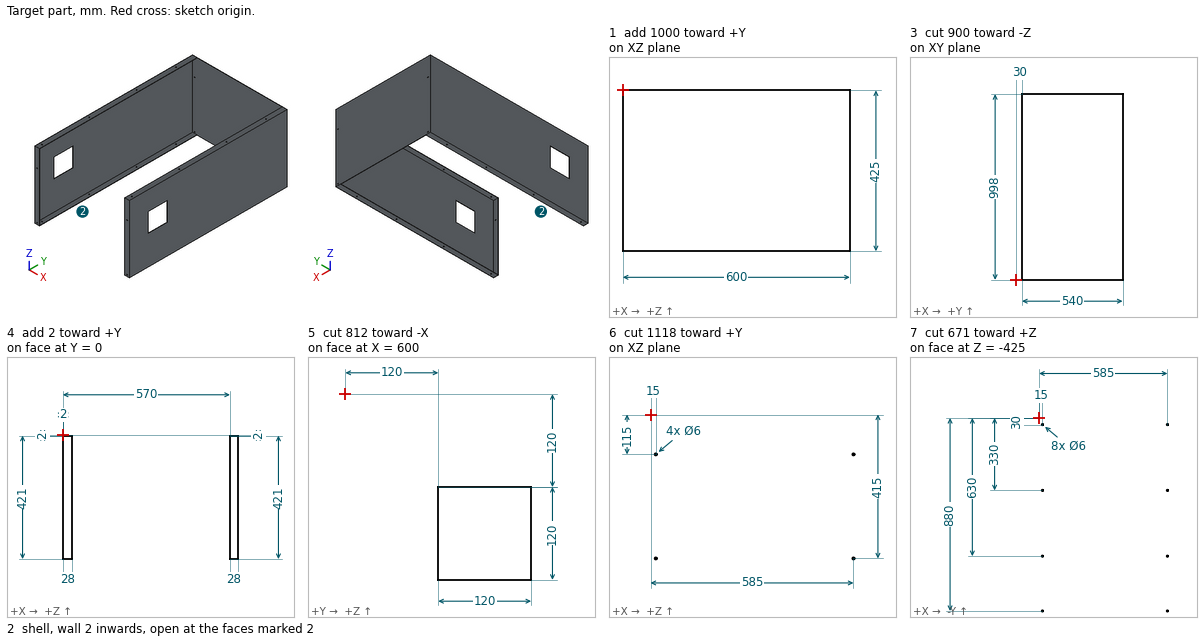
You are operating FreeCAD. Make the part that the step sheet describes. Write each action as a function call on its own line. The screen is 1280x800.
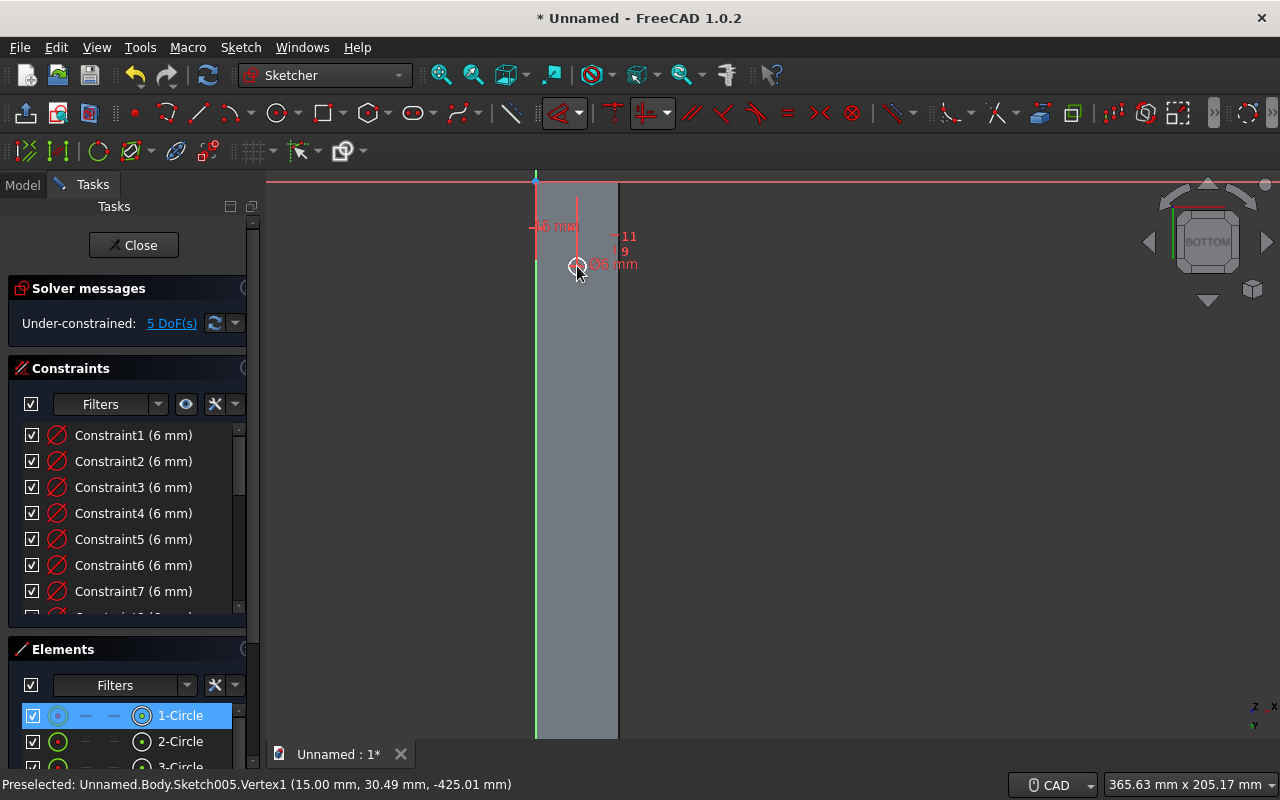
key(i)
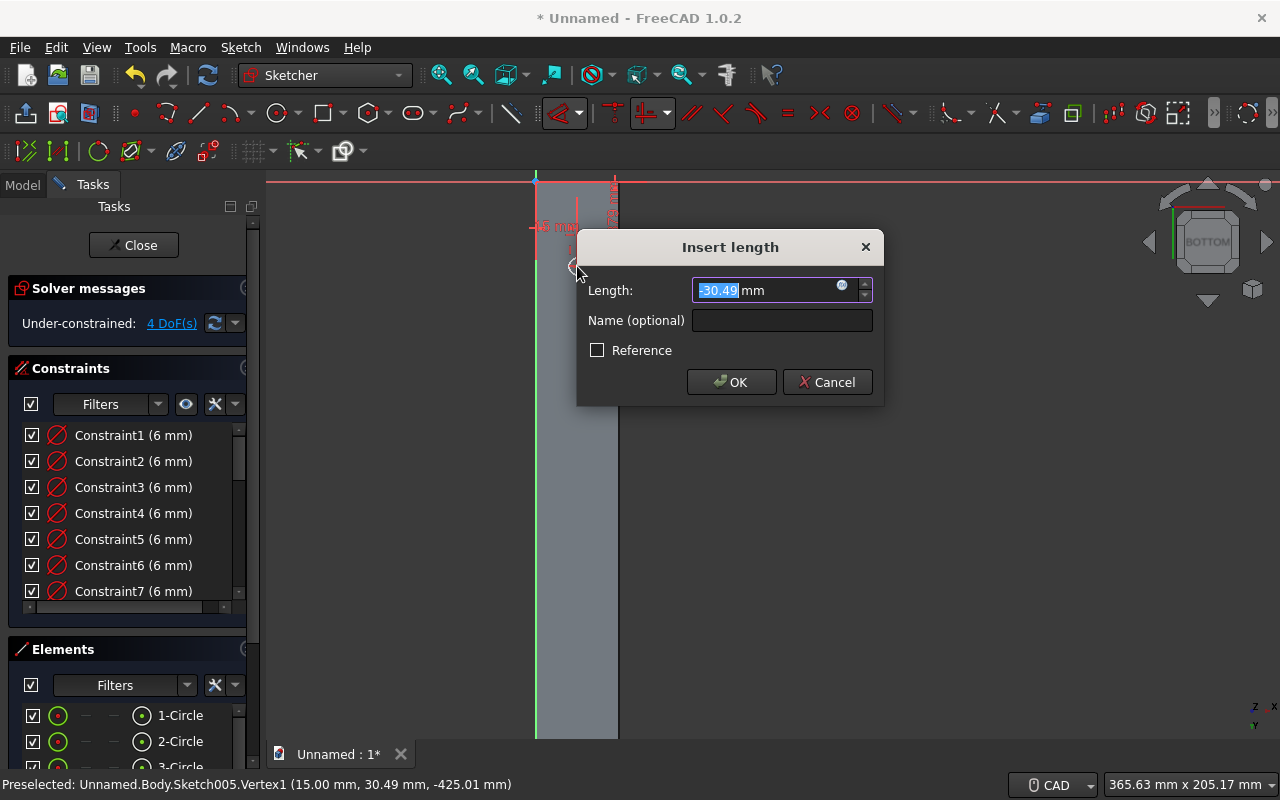
text(-30)
key(Return)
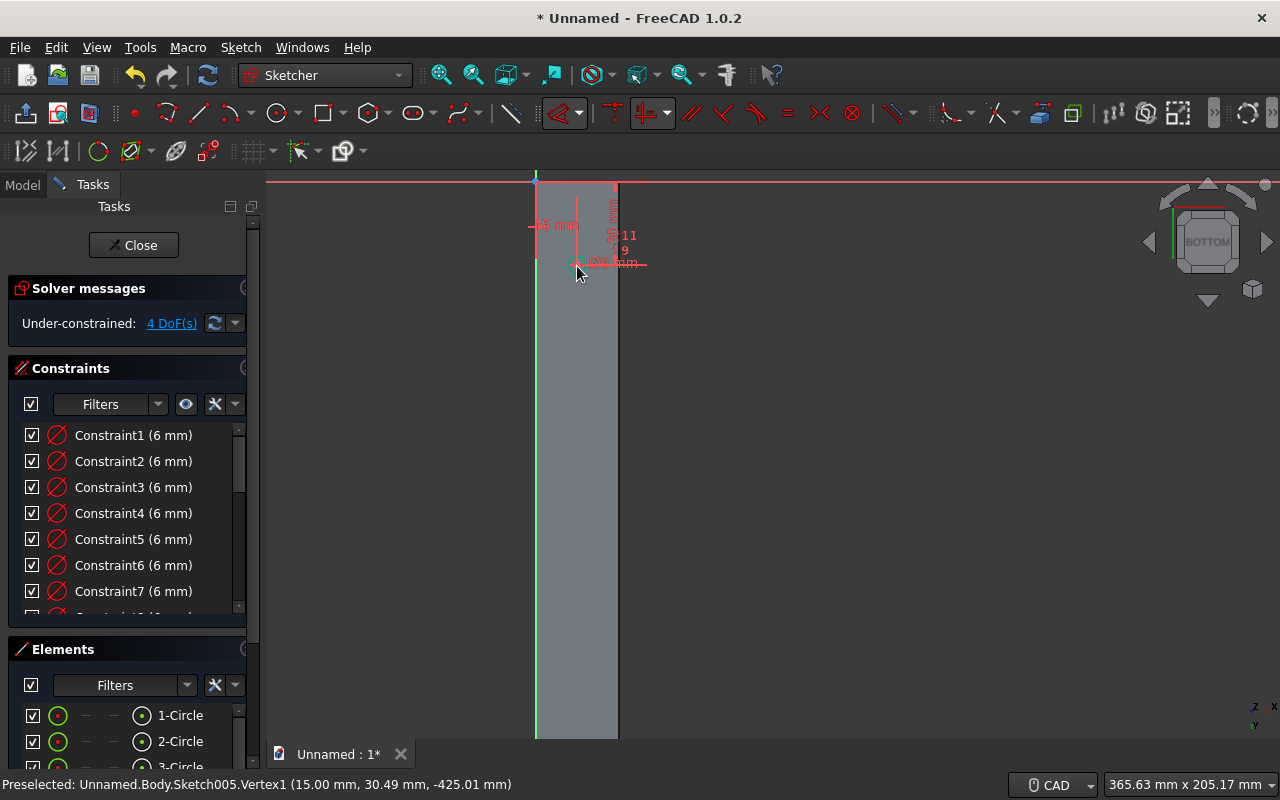
scroll(603, 306, down, 10)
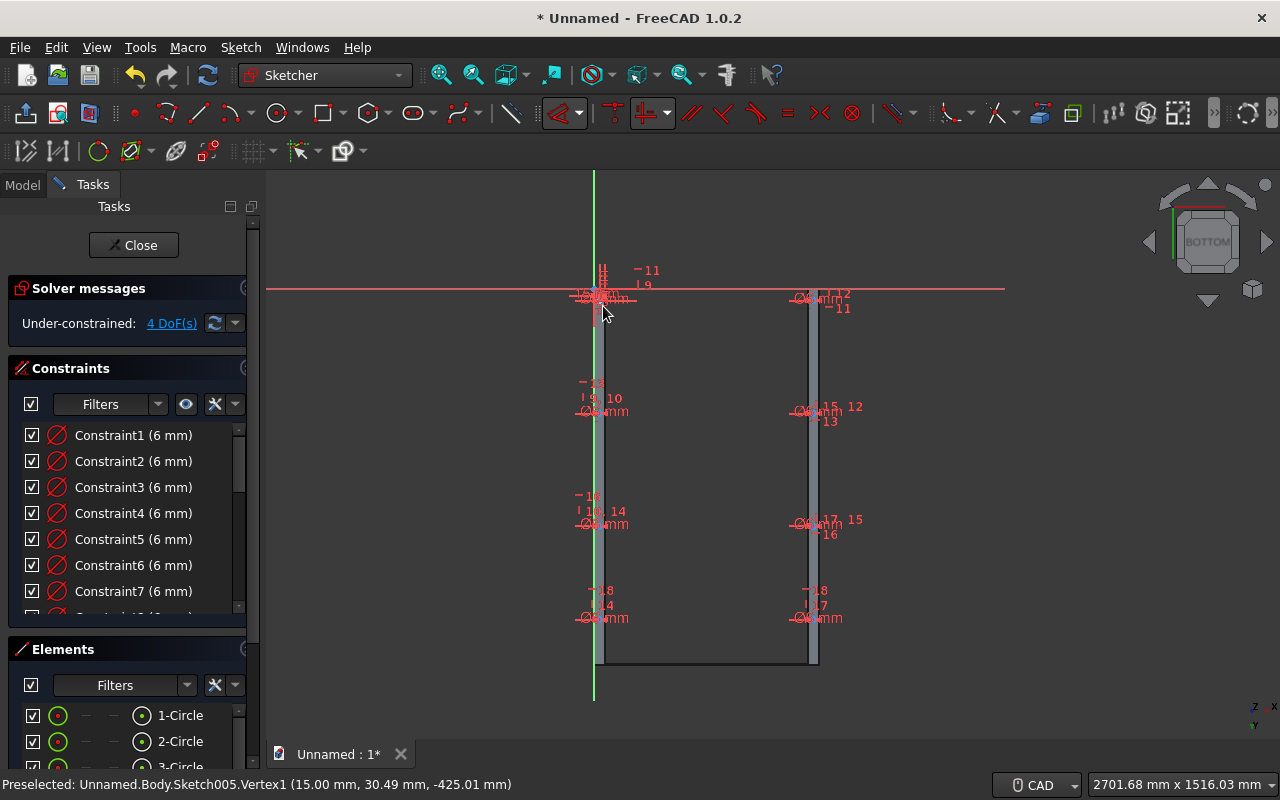
click(600, 414)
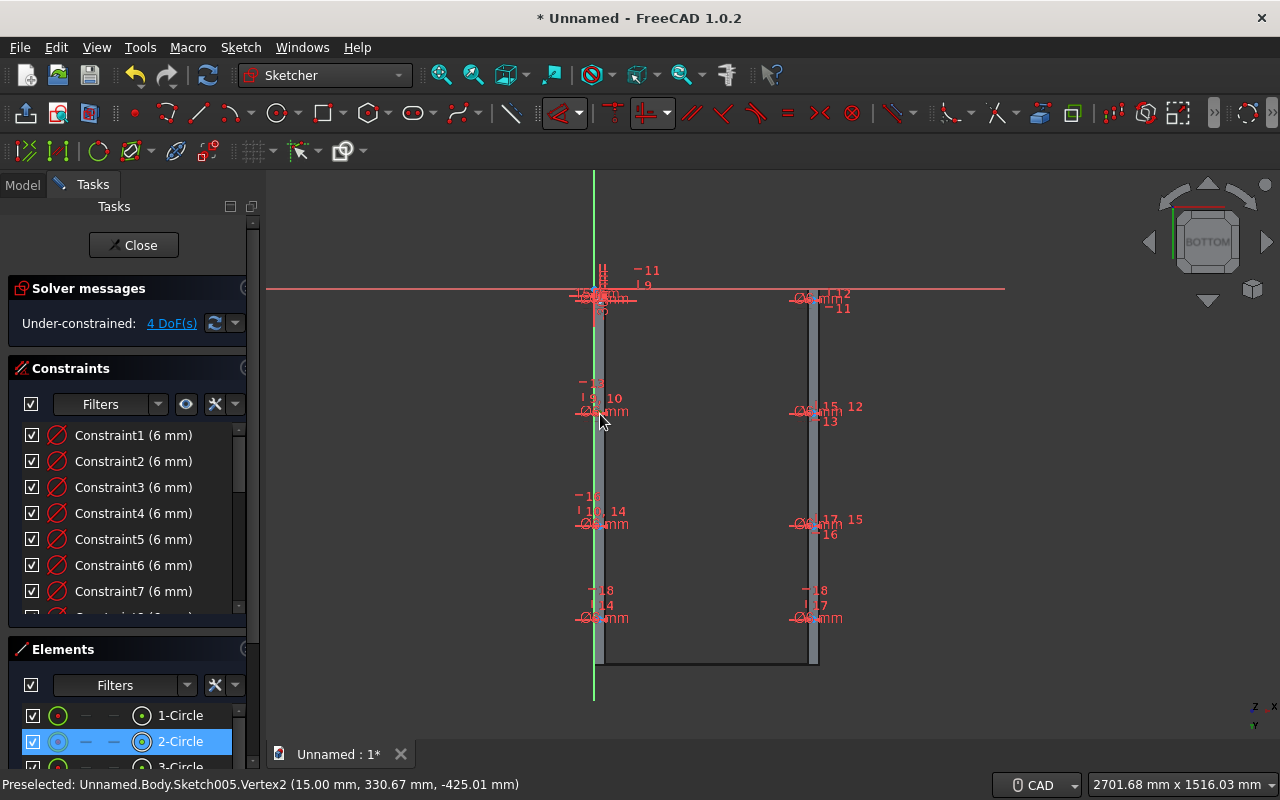
click(582, 114)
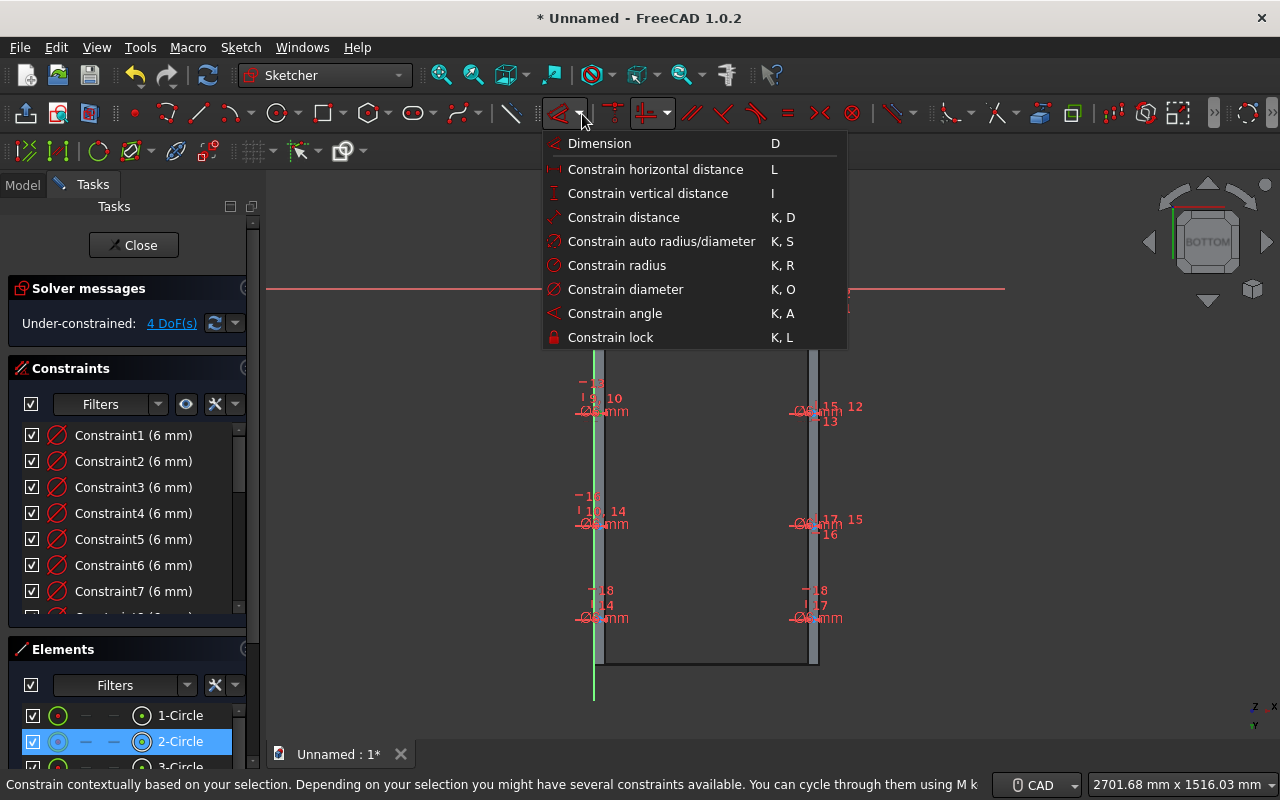
click(695, 193)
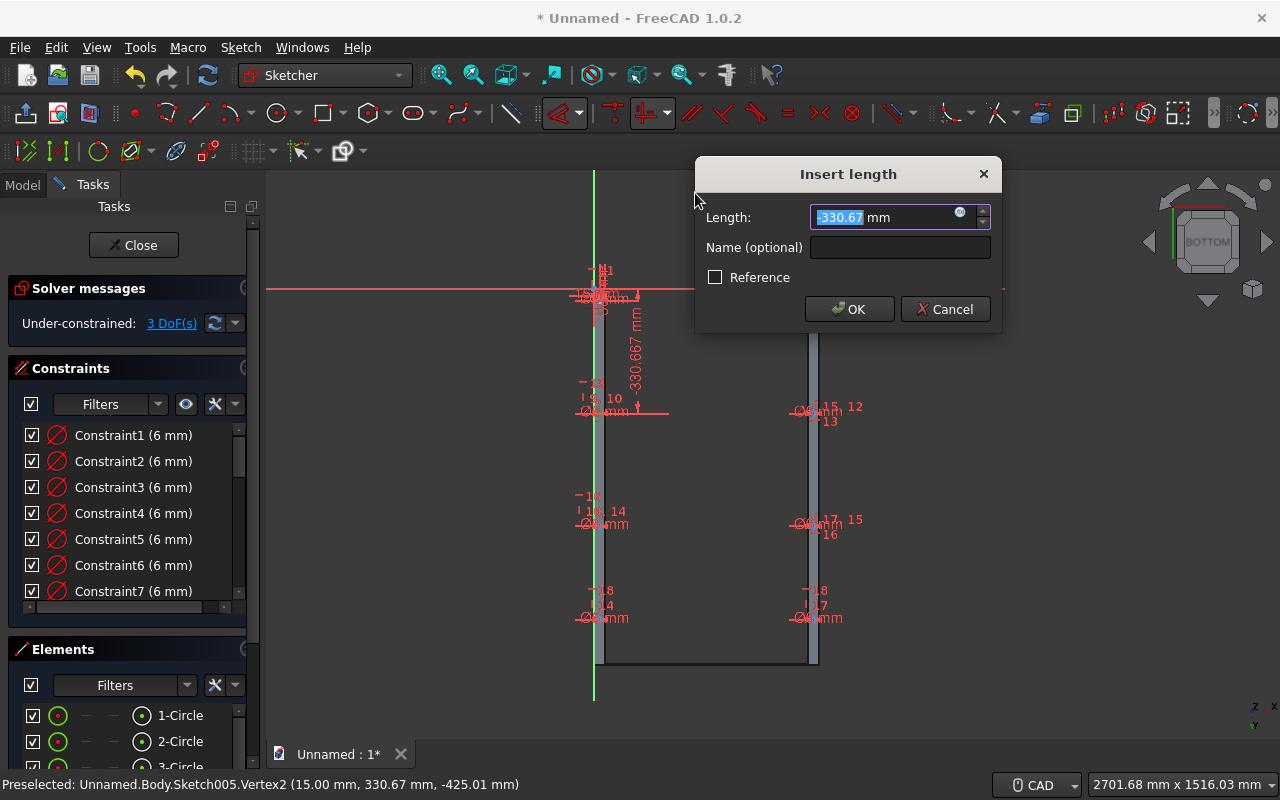
text(-330)
key(Return)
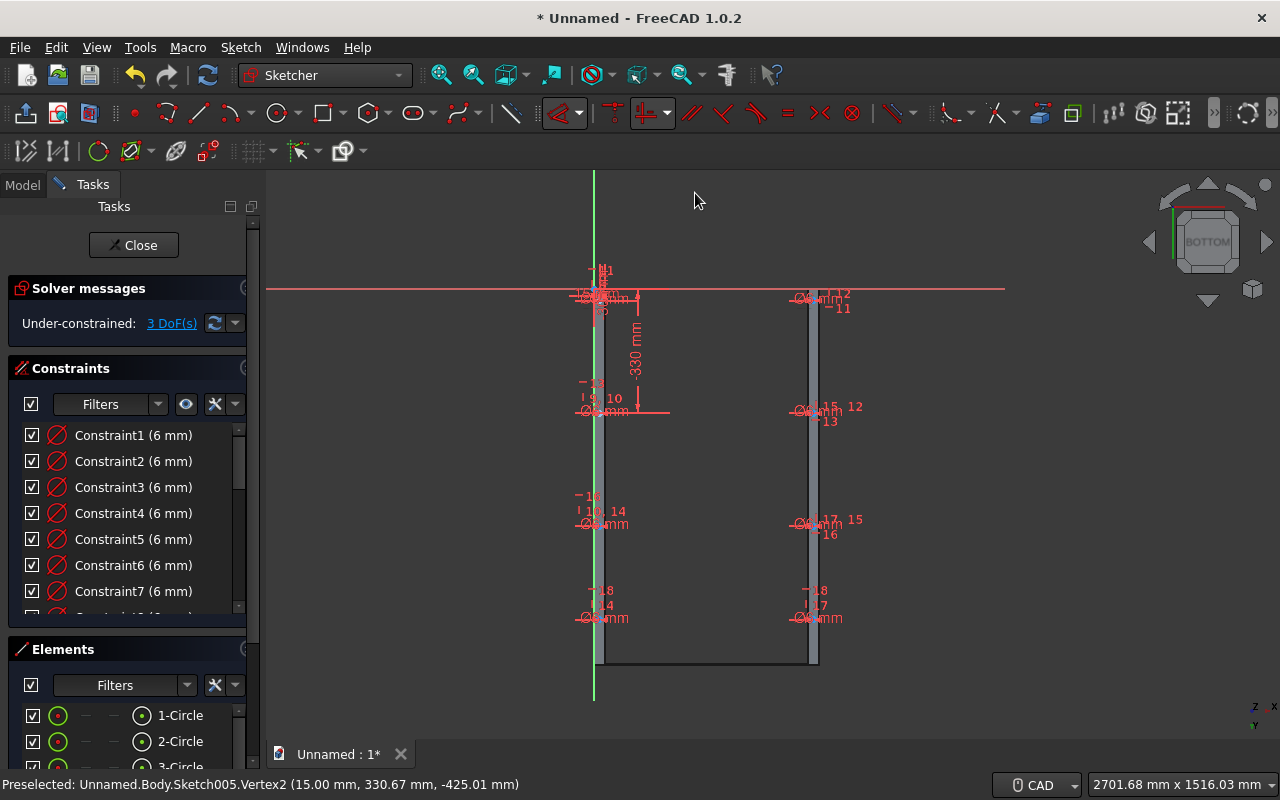
click(600, 526)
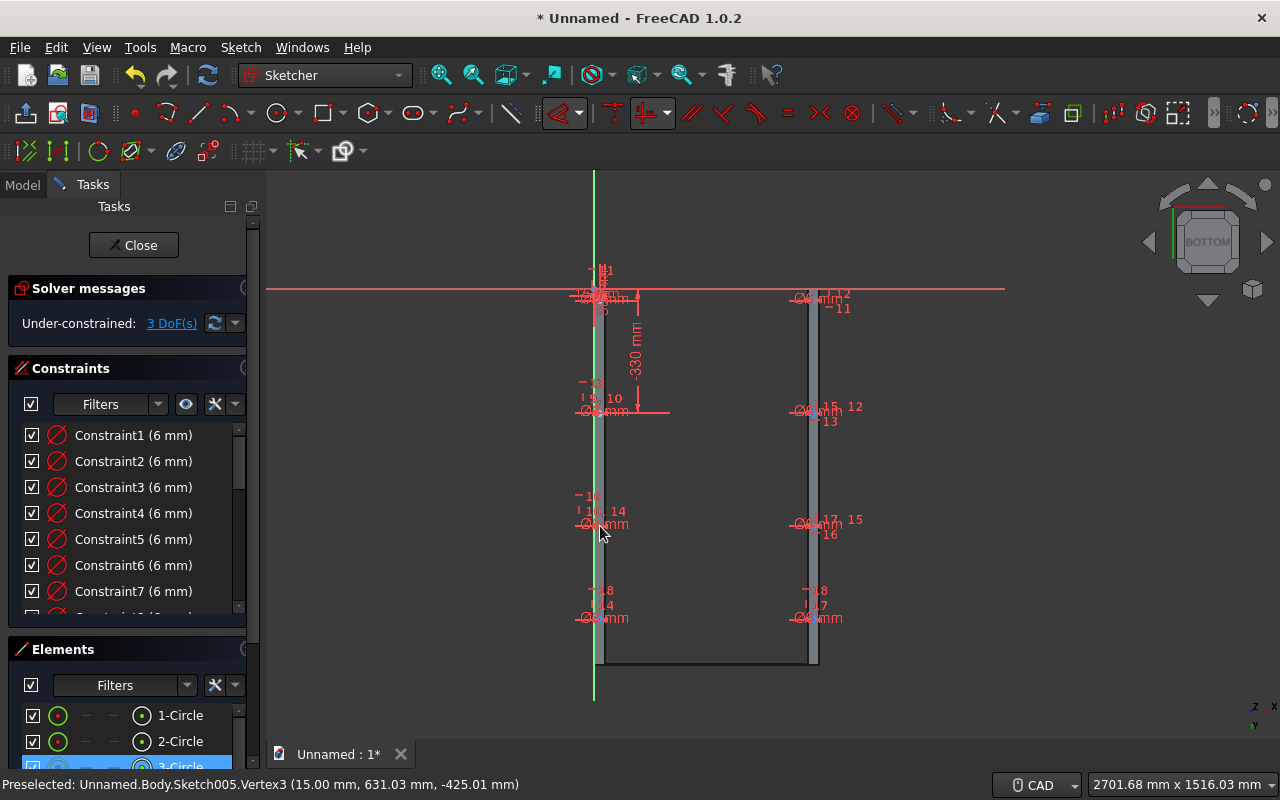
key(i)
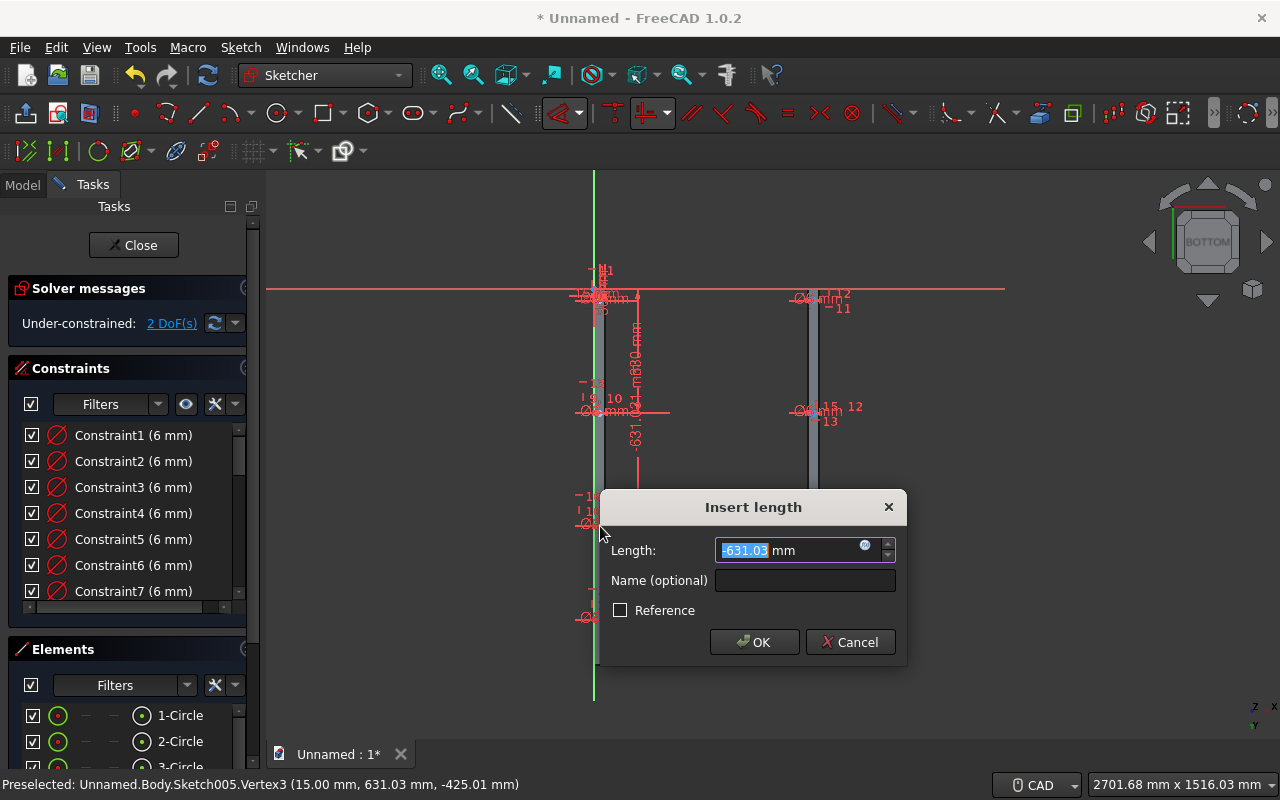
text(-630)
key(Return)